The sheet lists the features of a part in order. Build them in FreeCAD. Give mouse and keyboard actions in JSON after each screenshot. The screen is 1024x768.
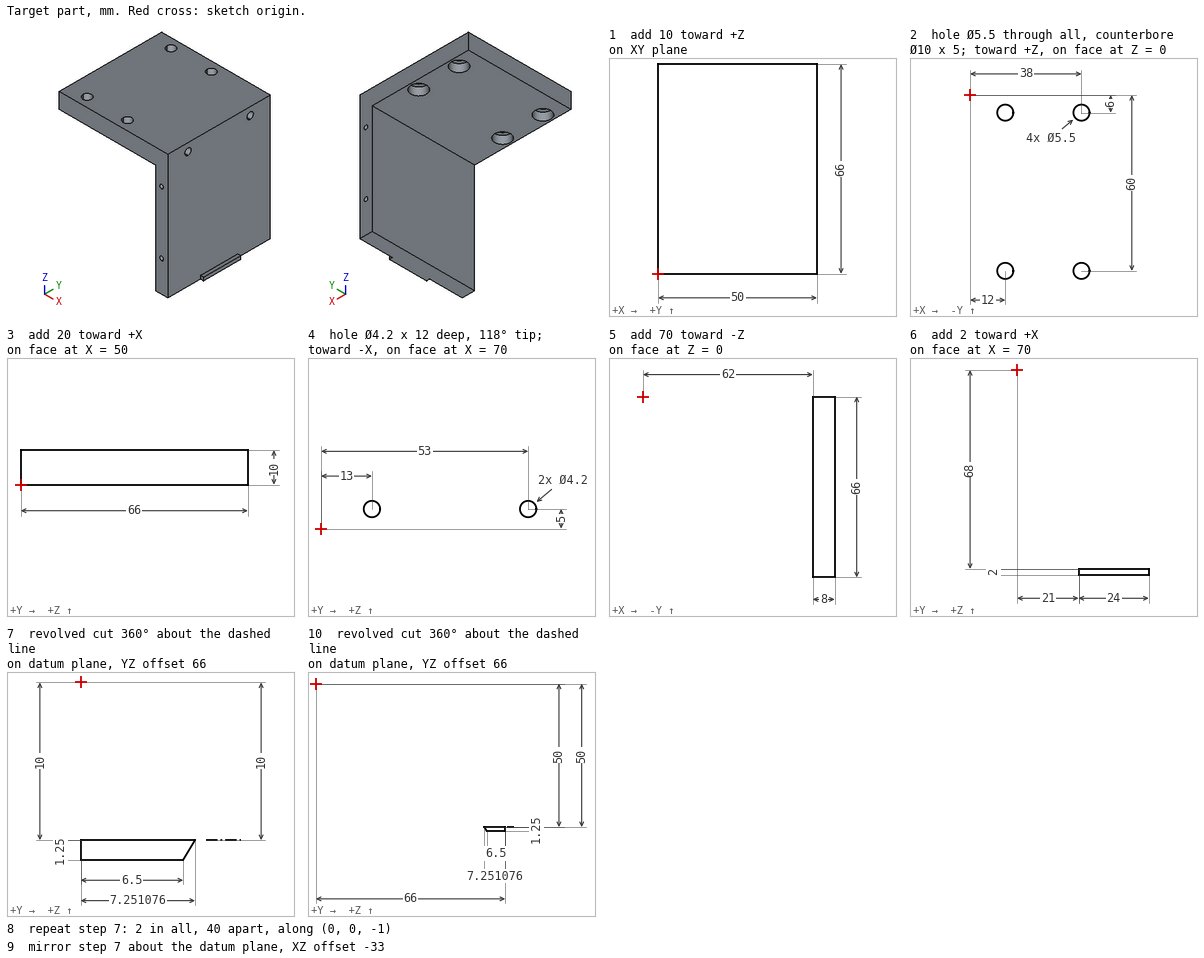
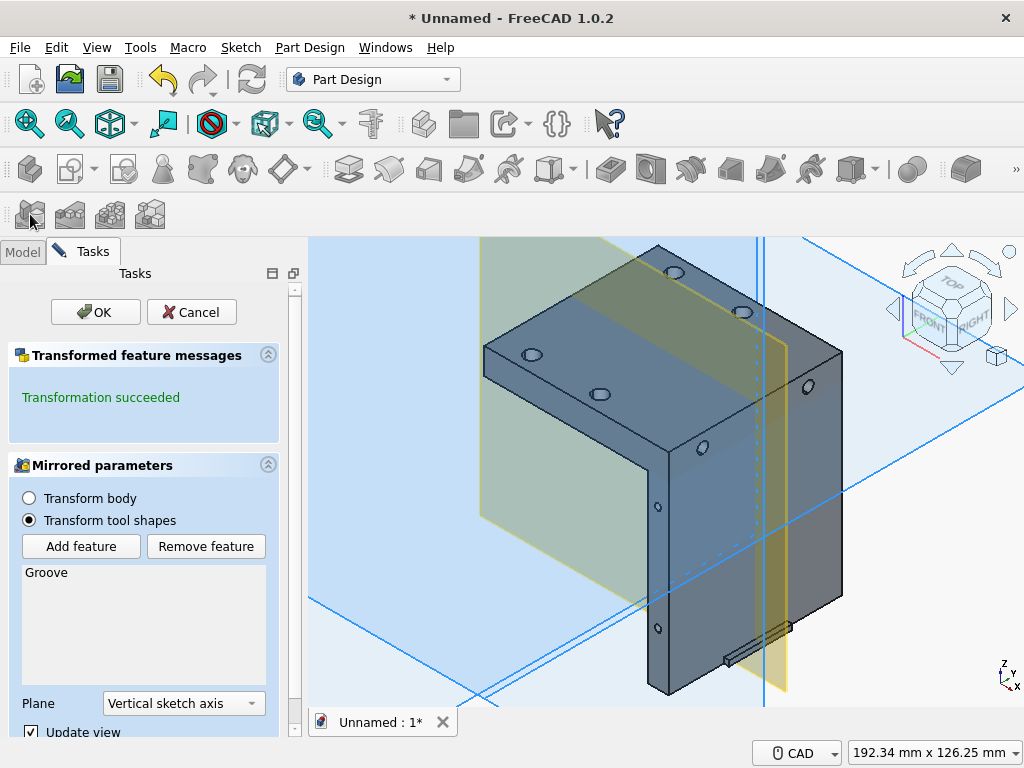
{"action": "left_click", "coordinate": [184, 704]}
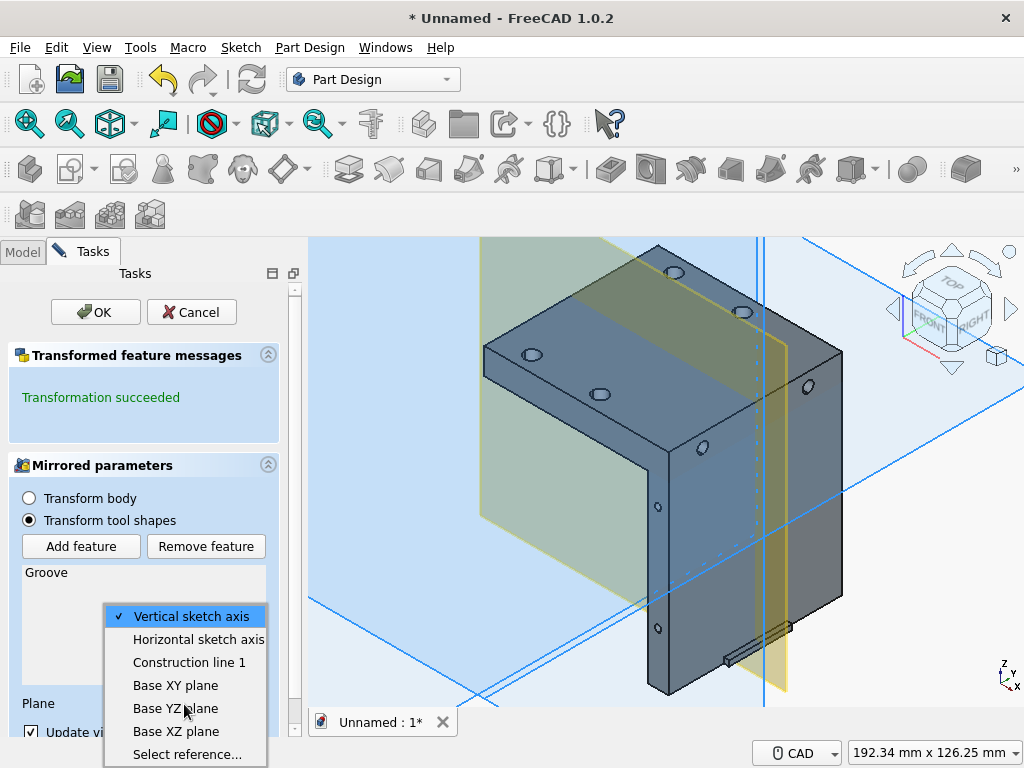
{"action": "left_click", "coordinate": [184, 754]}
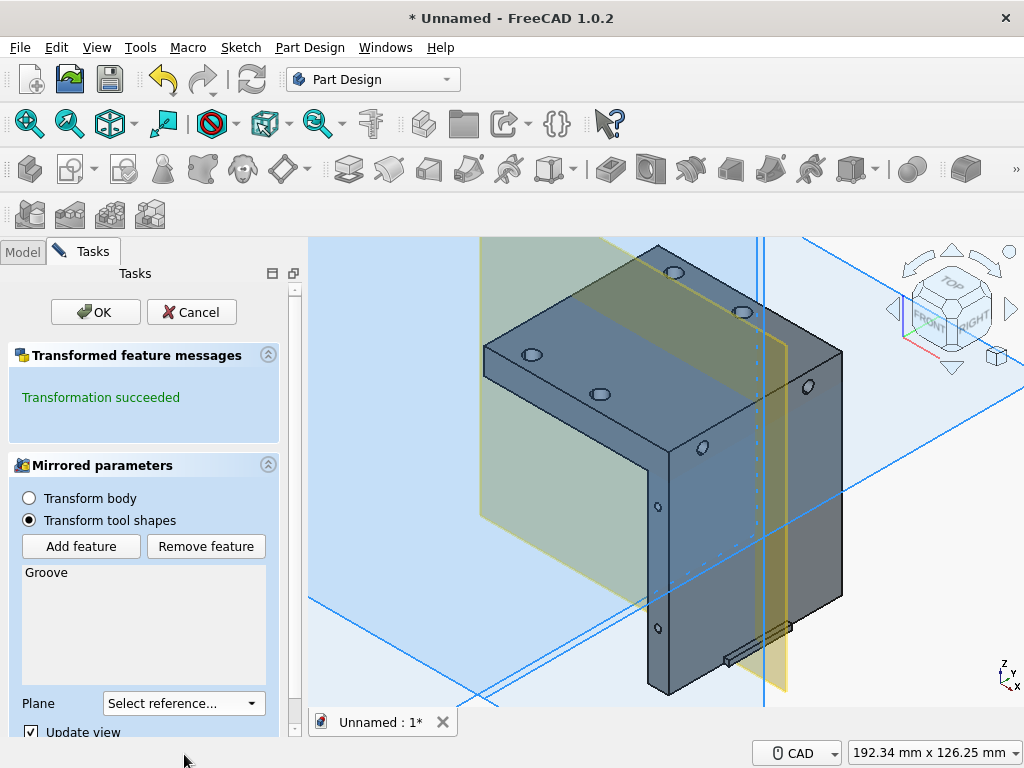
{"action": "left_click", "coordinate": [23, 251]}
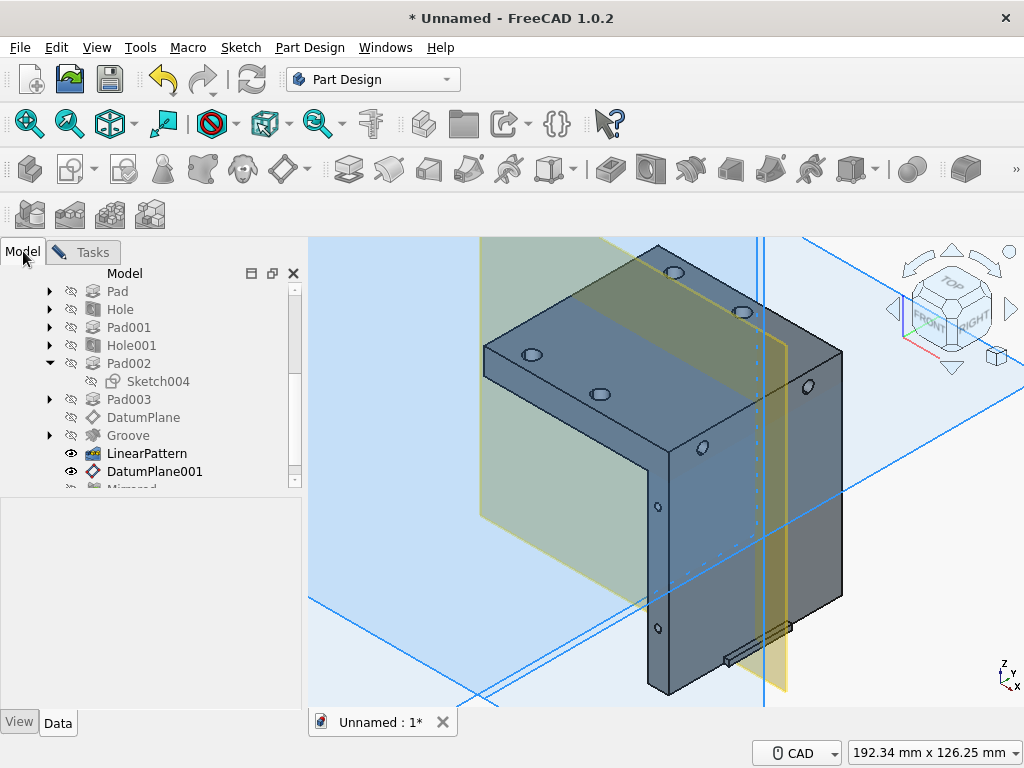
{"action": "left_click", "coordinate": [116, 471]}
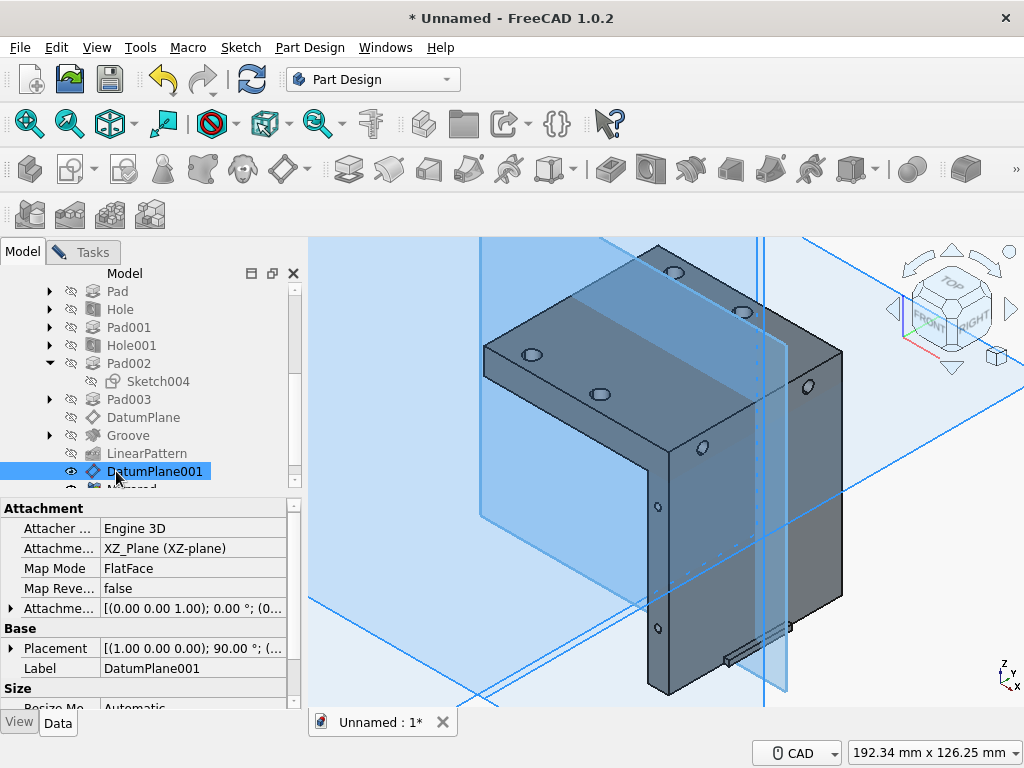
{"action": "left_click", "coordinate": [84, 251]}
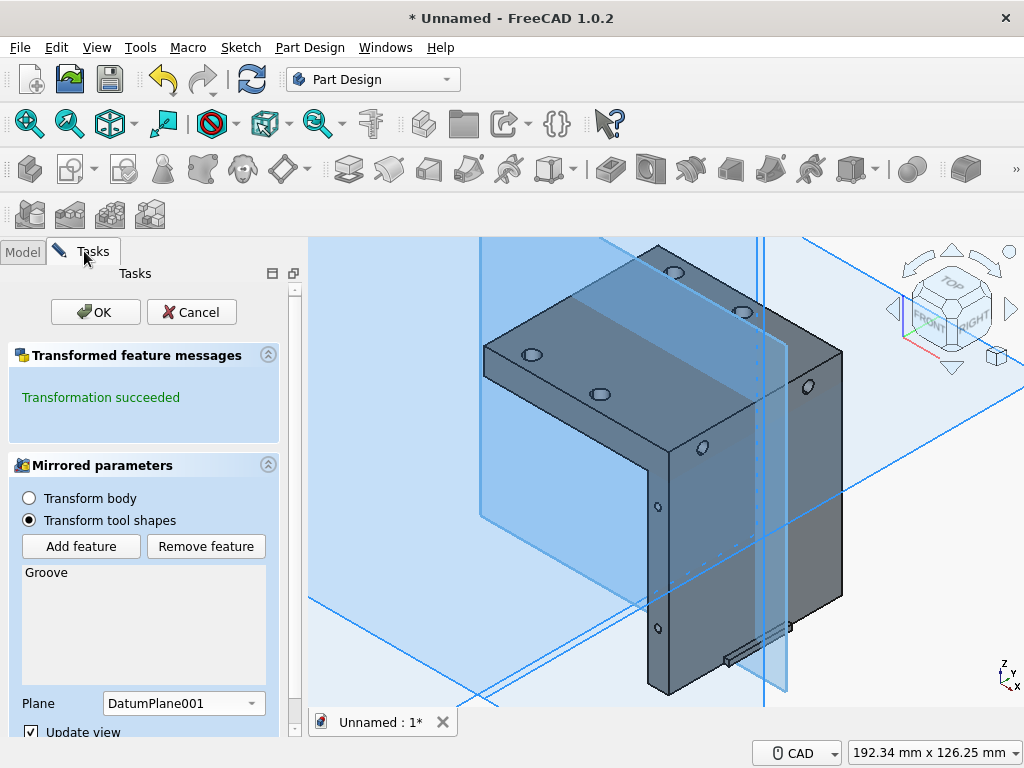
{"action": "left_click", "coordinate": [96, 312]}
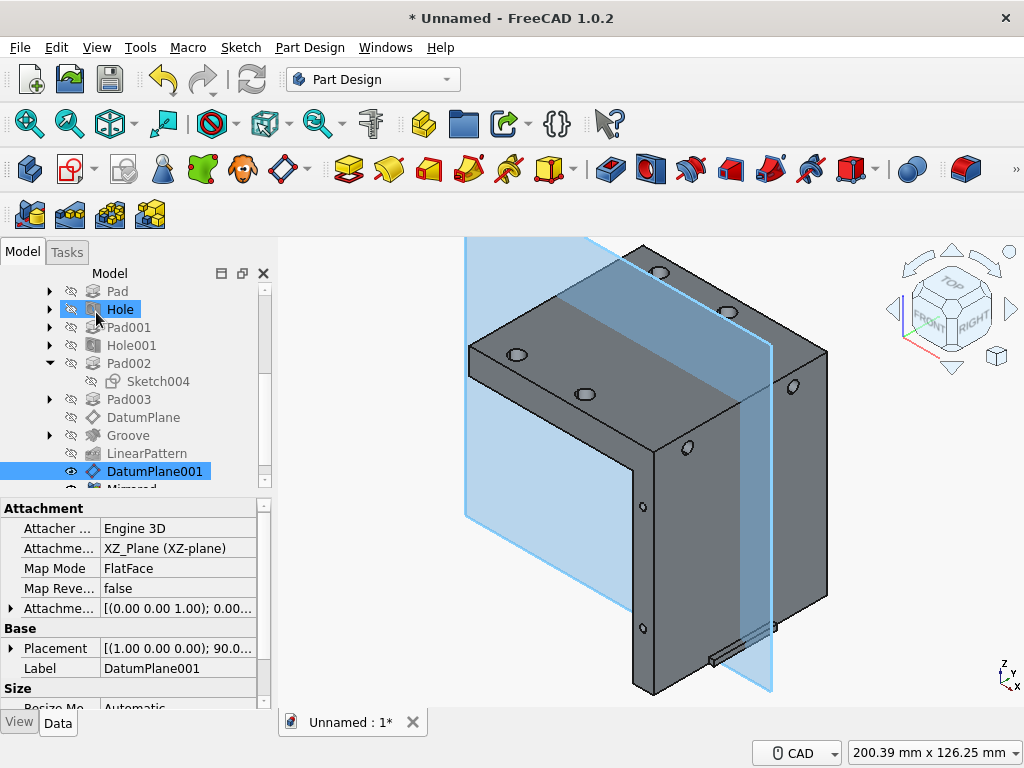
{"action": "left_click", "coordinate": [116, 471]}
{"action": "key", "text": "space"}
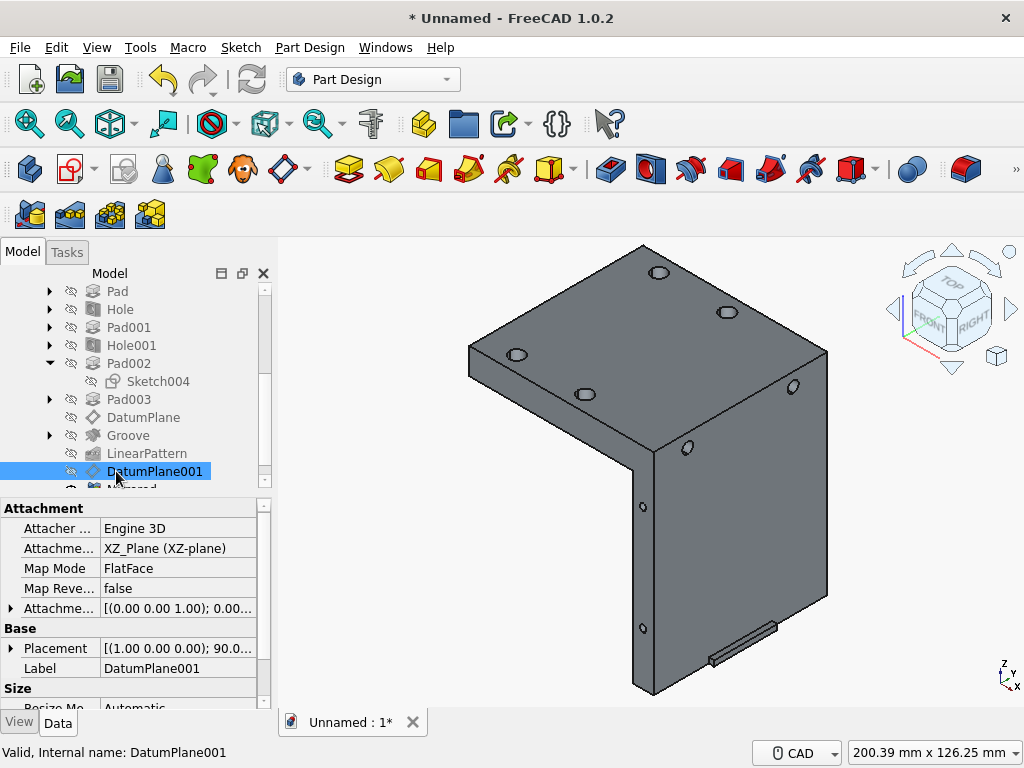
{"action": "scroll", "coordinate": [140, 377], "scroll_direction": "down", "scroll_amount": 3}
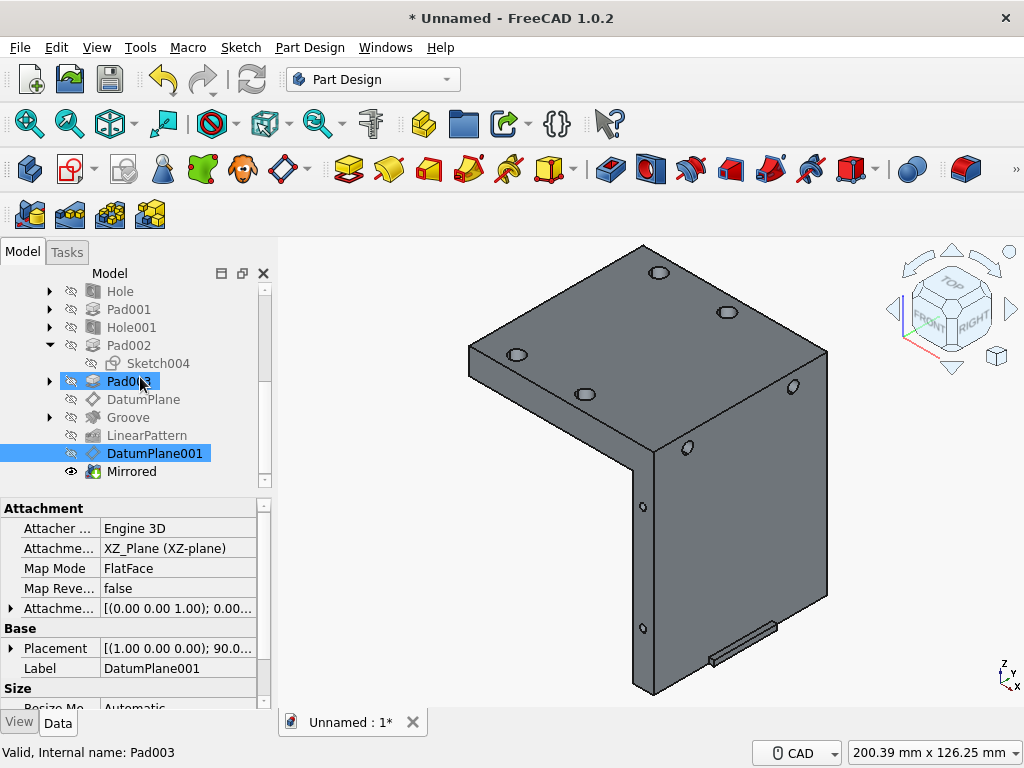
{"action": "scroll", "coordinate": [140, 377], "scroll_direction": "up", "scroll_amount": 15}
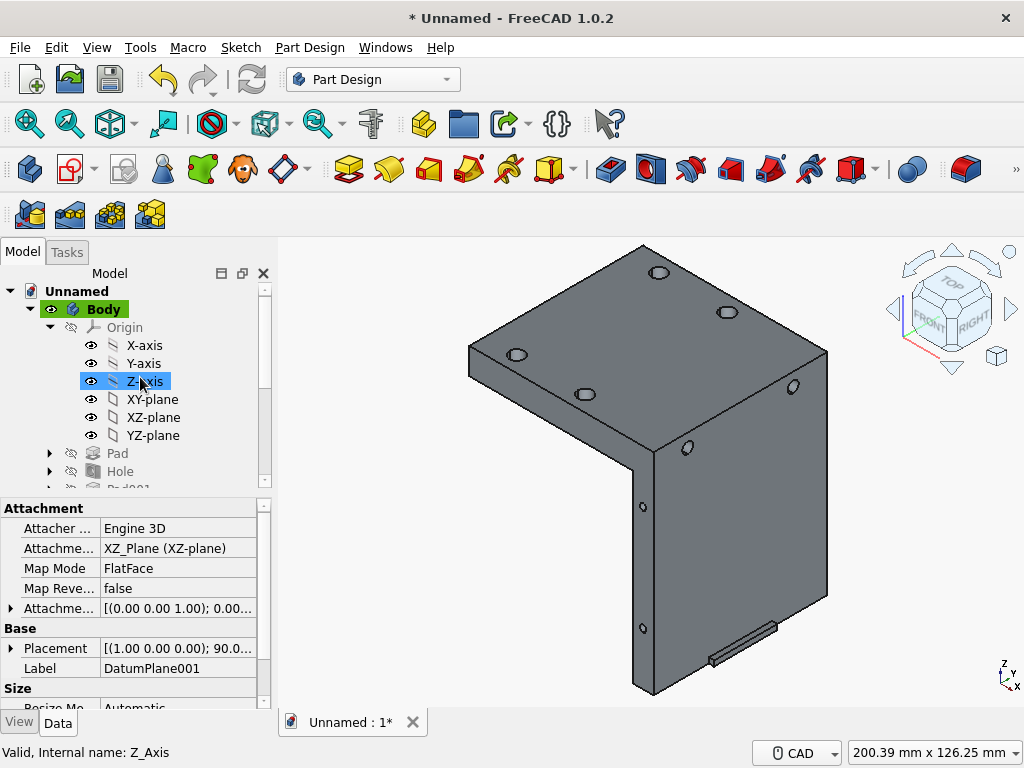
{"action": "left_click", "coordinate": [136, 435]}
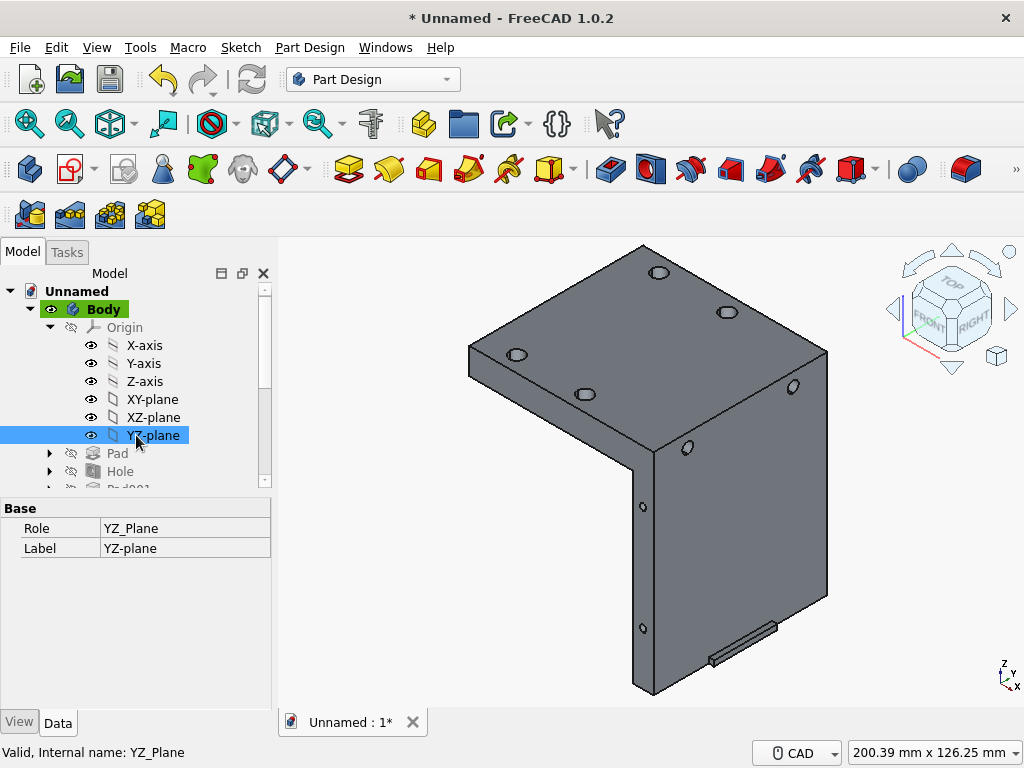
{"action": "left_click", "coordinate": [284, 170]}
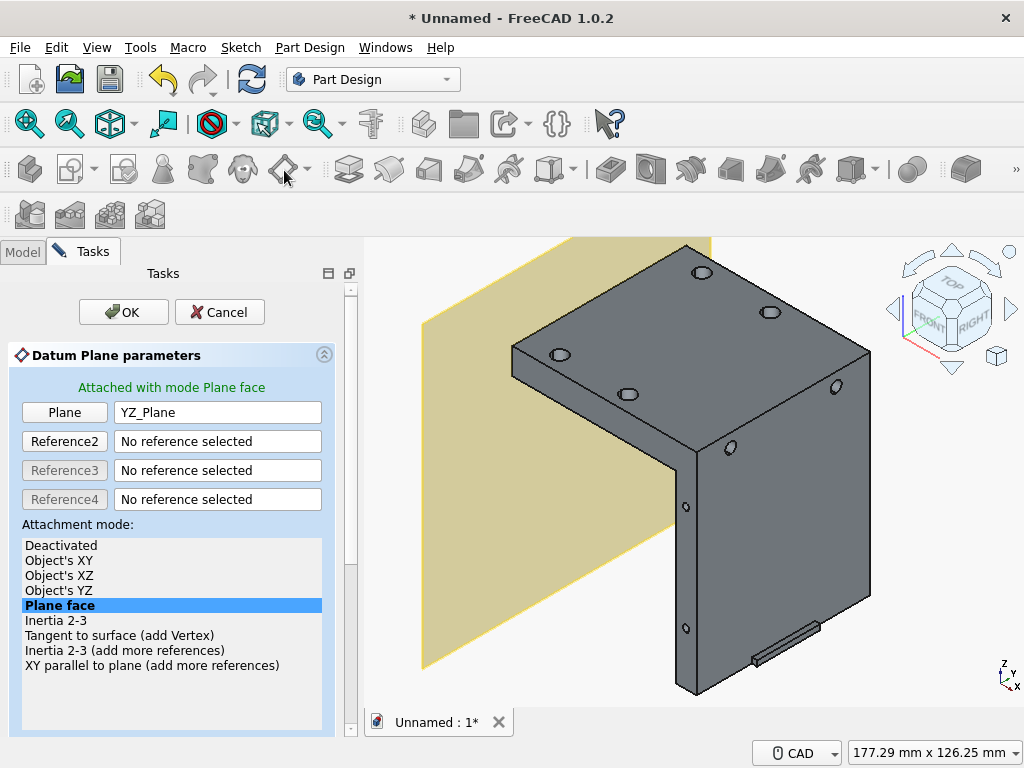
{"action": "scroll", "coordinate": [351, 510], "scroll_direction": "down", "scroll_amount": 3}